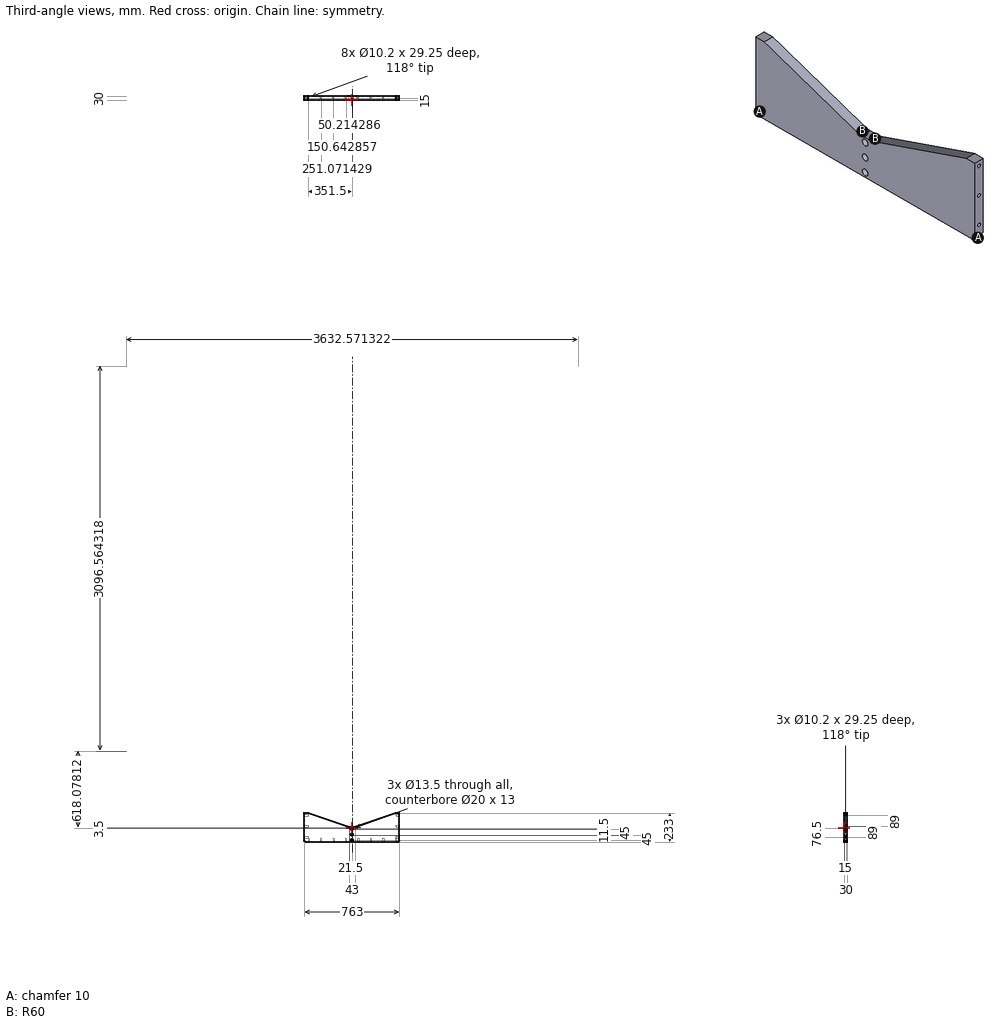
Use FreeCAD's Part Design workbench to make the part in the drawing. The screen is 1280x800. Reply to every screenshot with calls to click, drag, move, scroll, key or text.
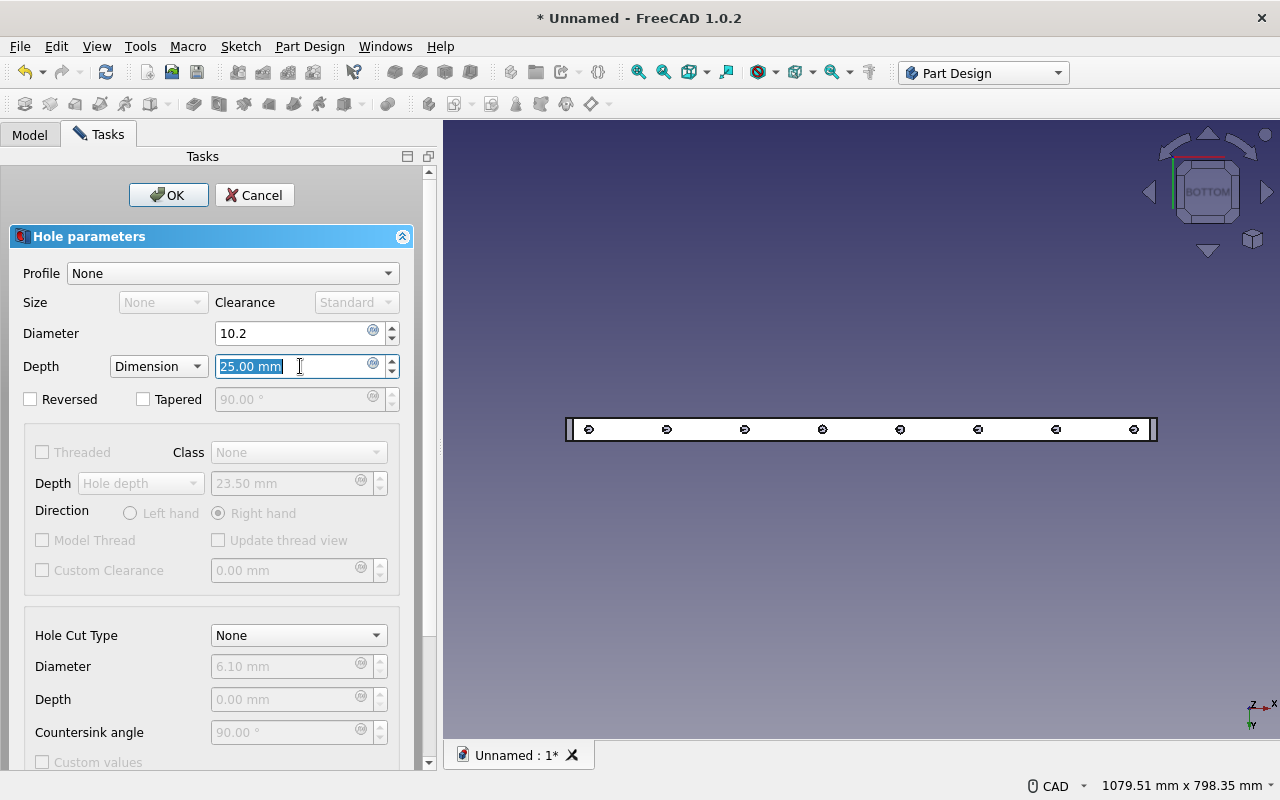
text(29.25)
key(Tab)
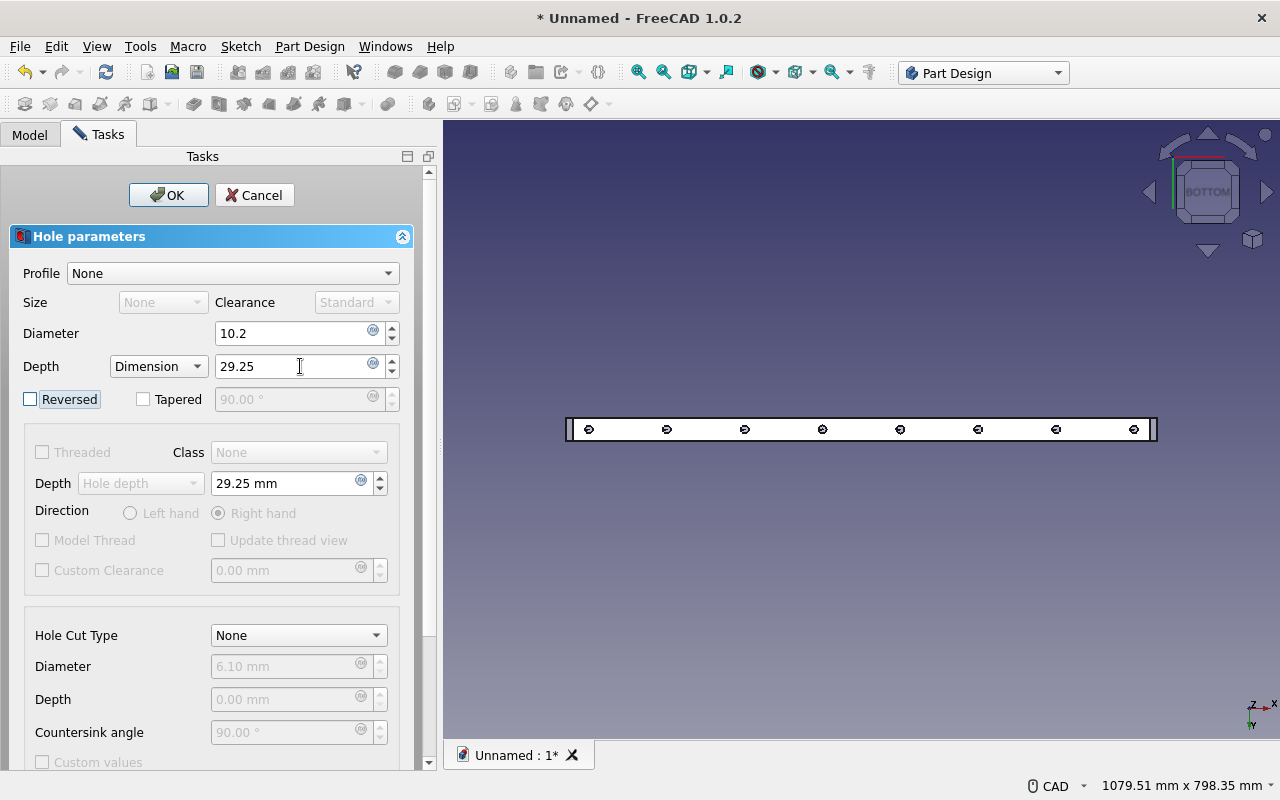
click(169, 195)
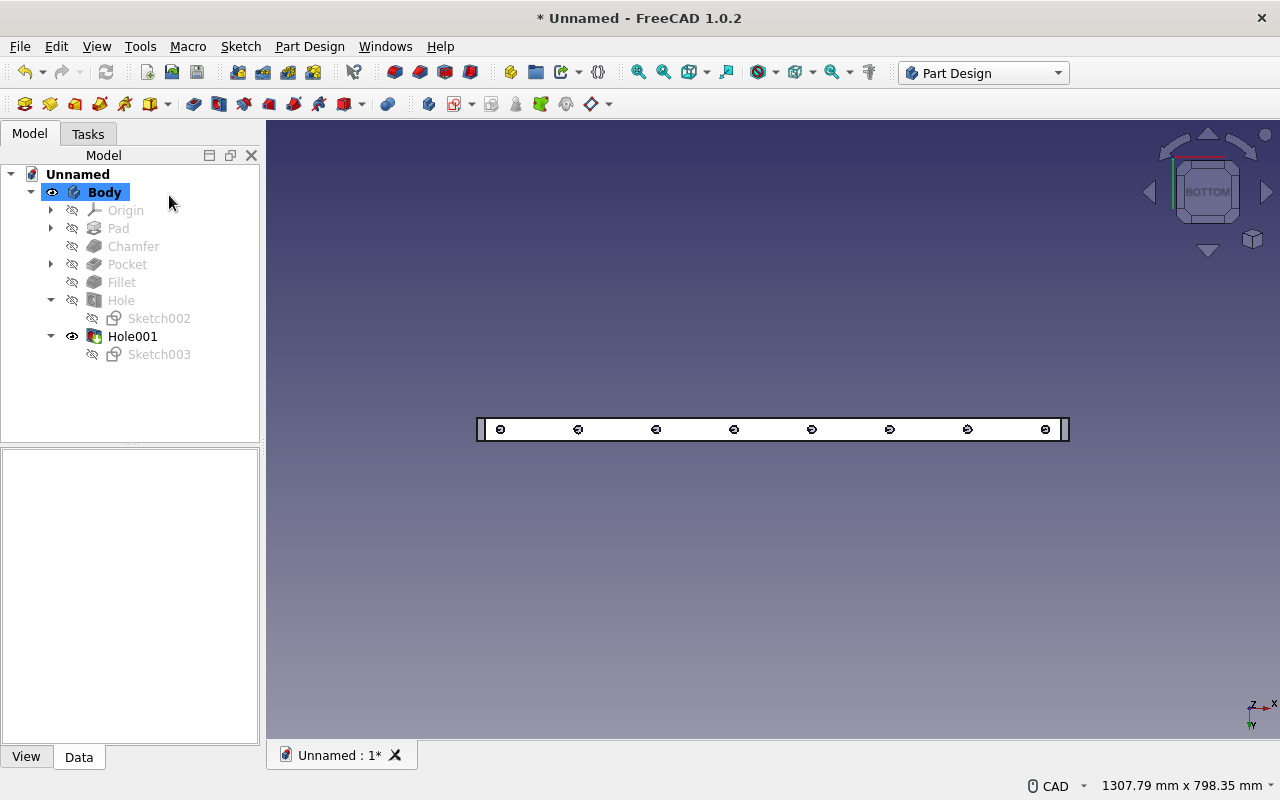
key(6)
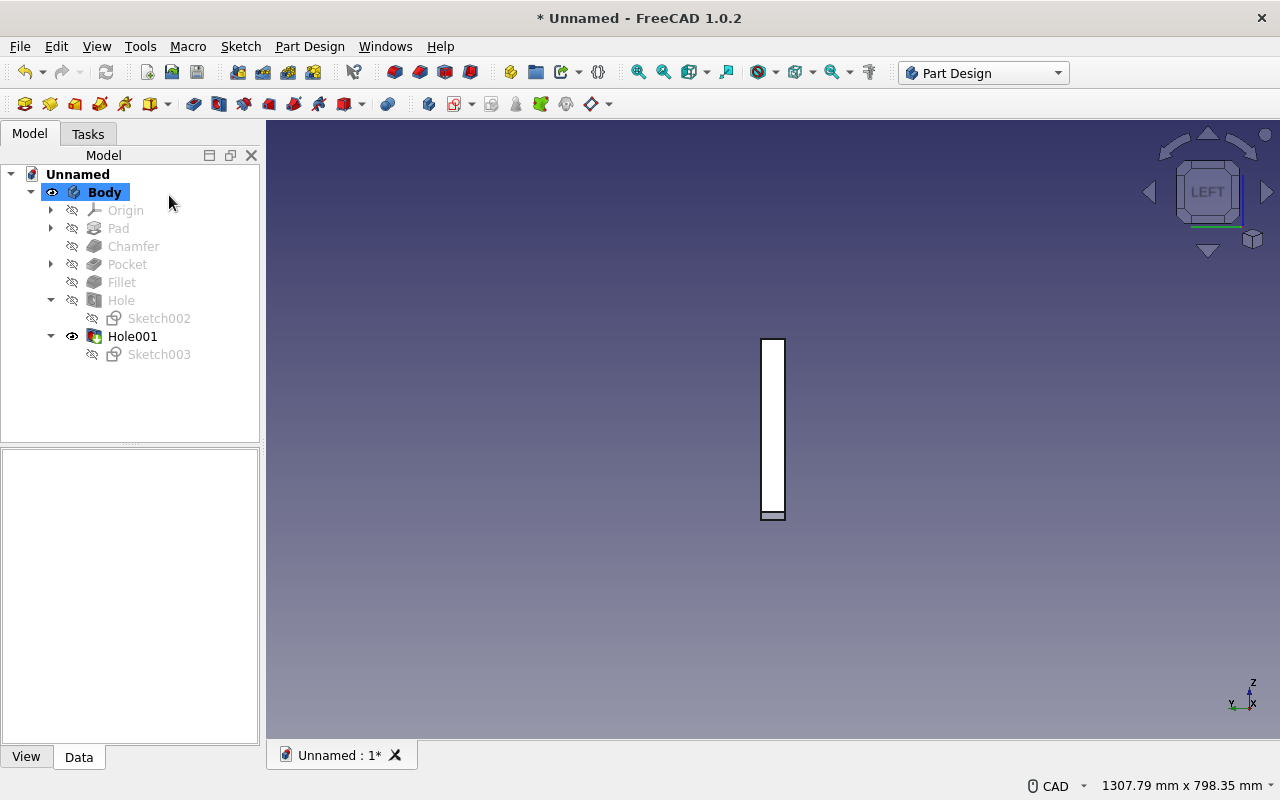
key(v)
key(f)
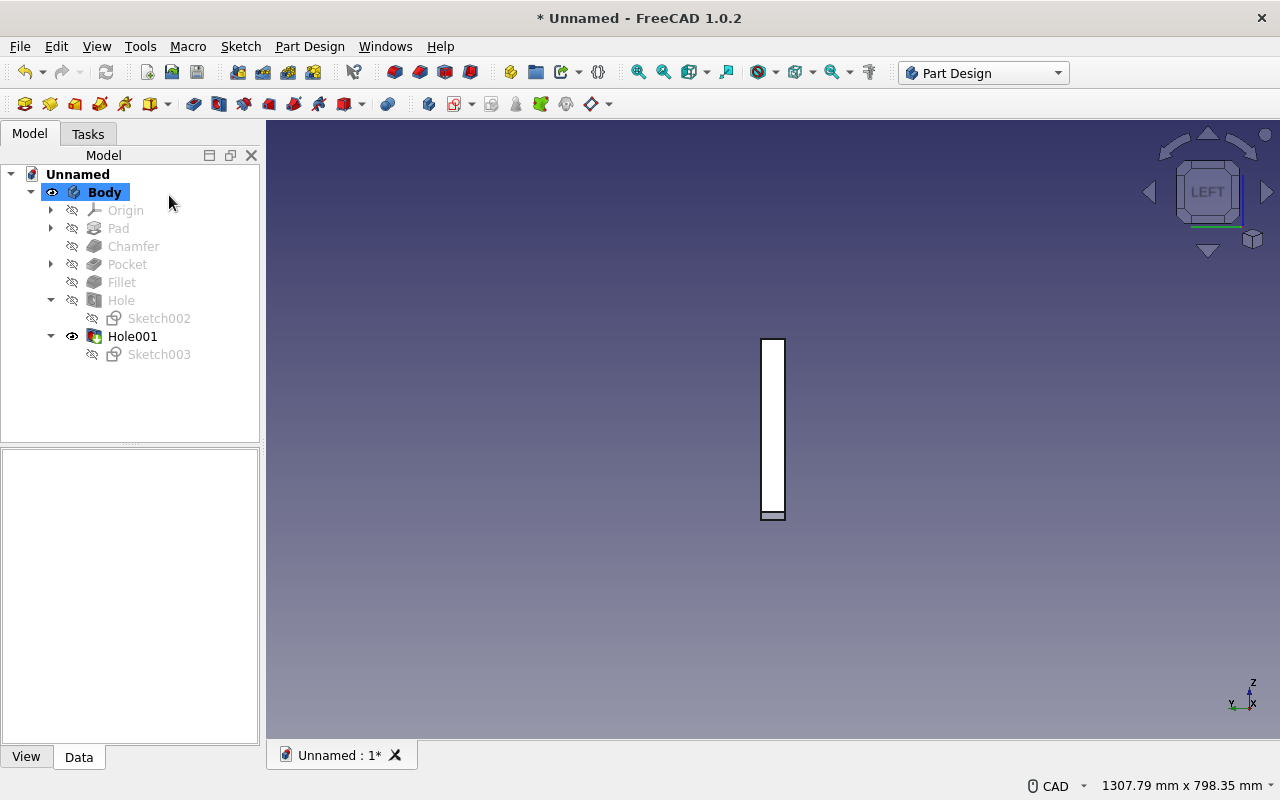
click(773, 474)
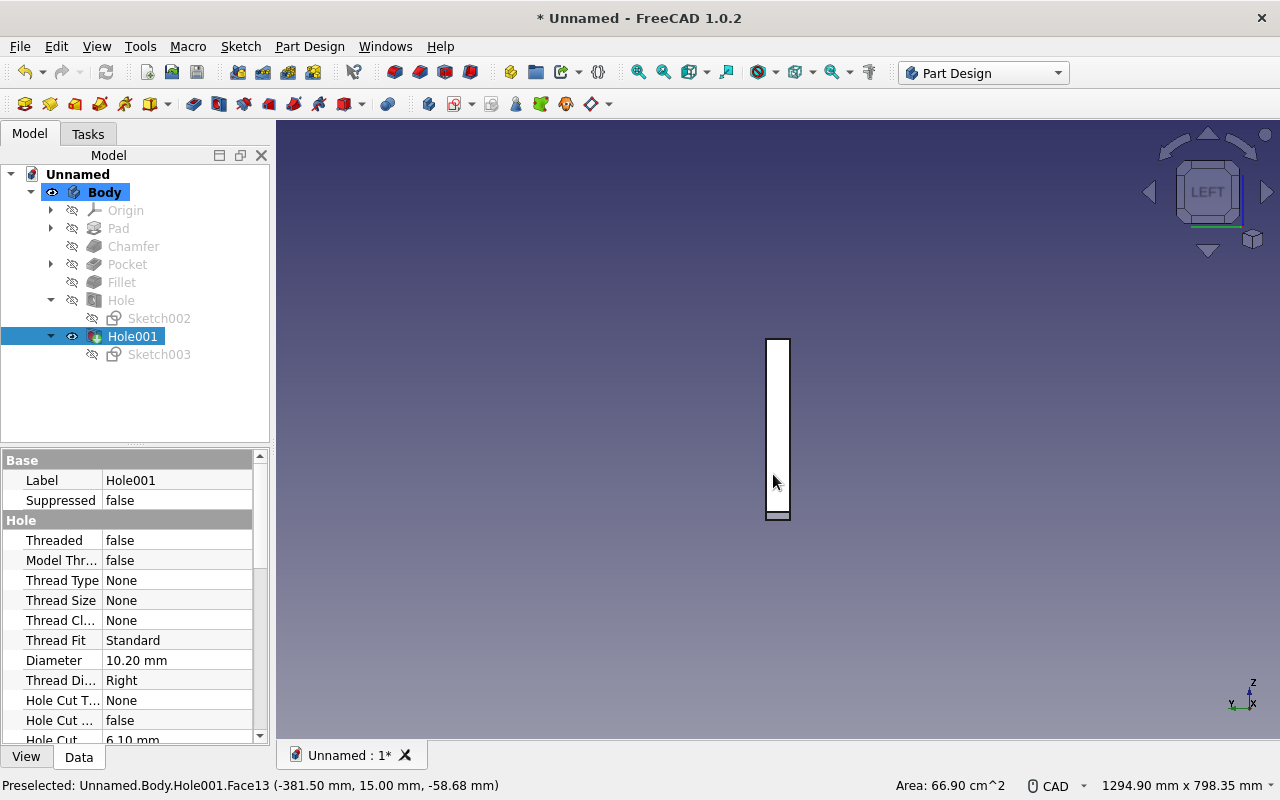
click(454, 104)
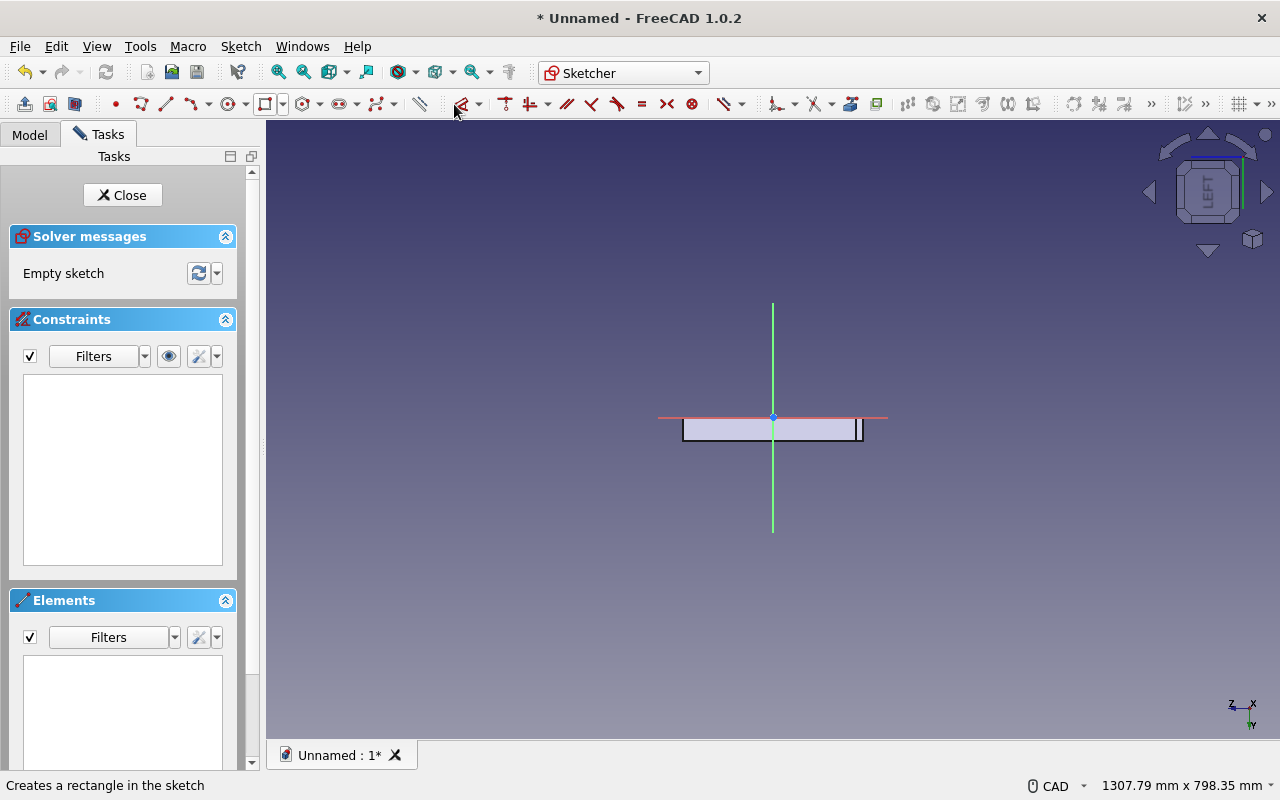
scroll(783, 424, up, 7)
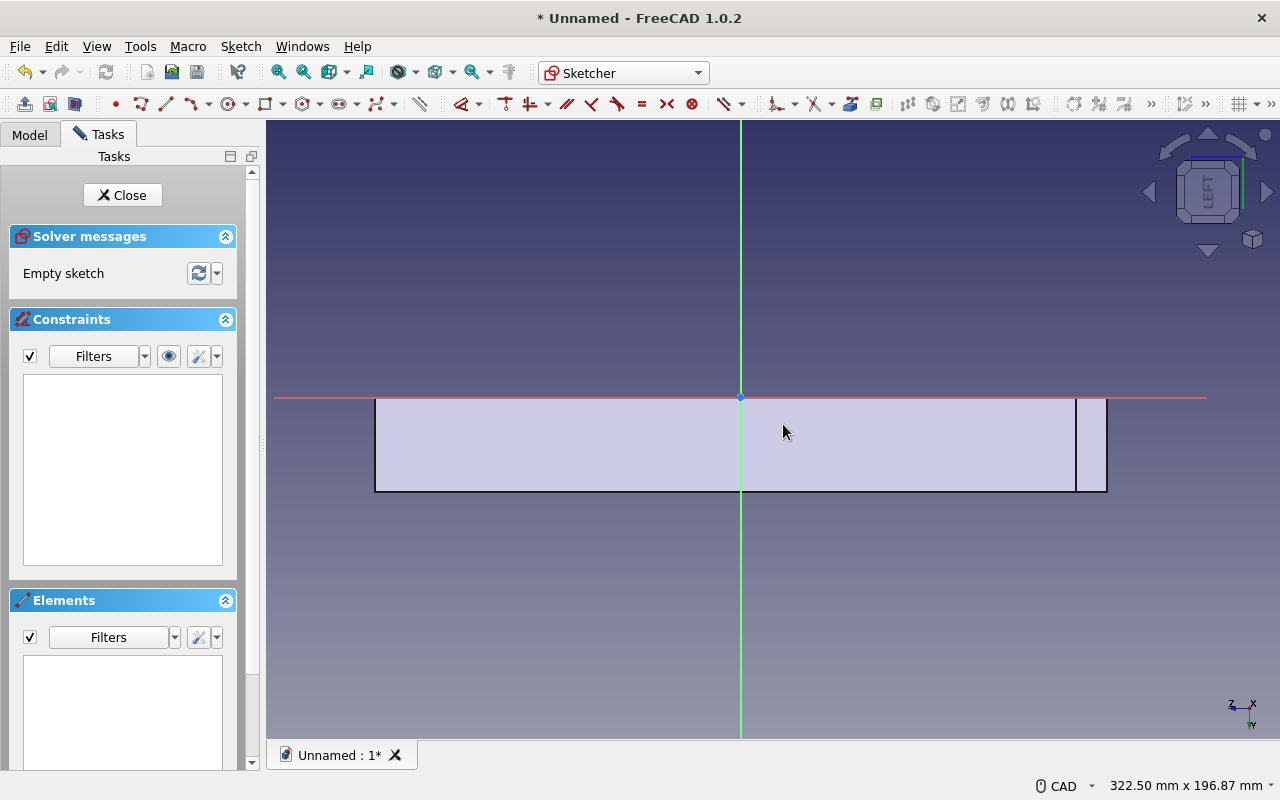
key(g)
key(c)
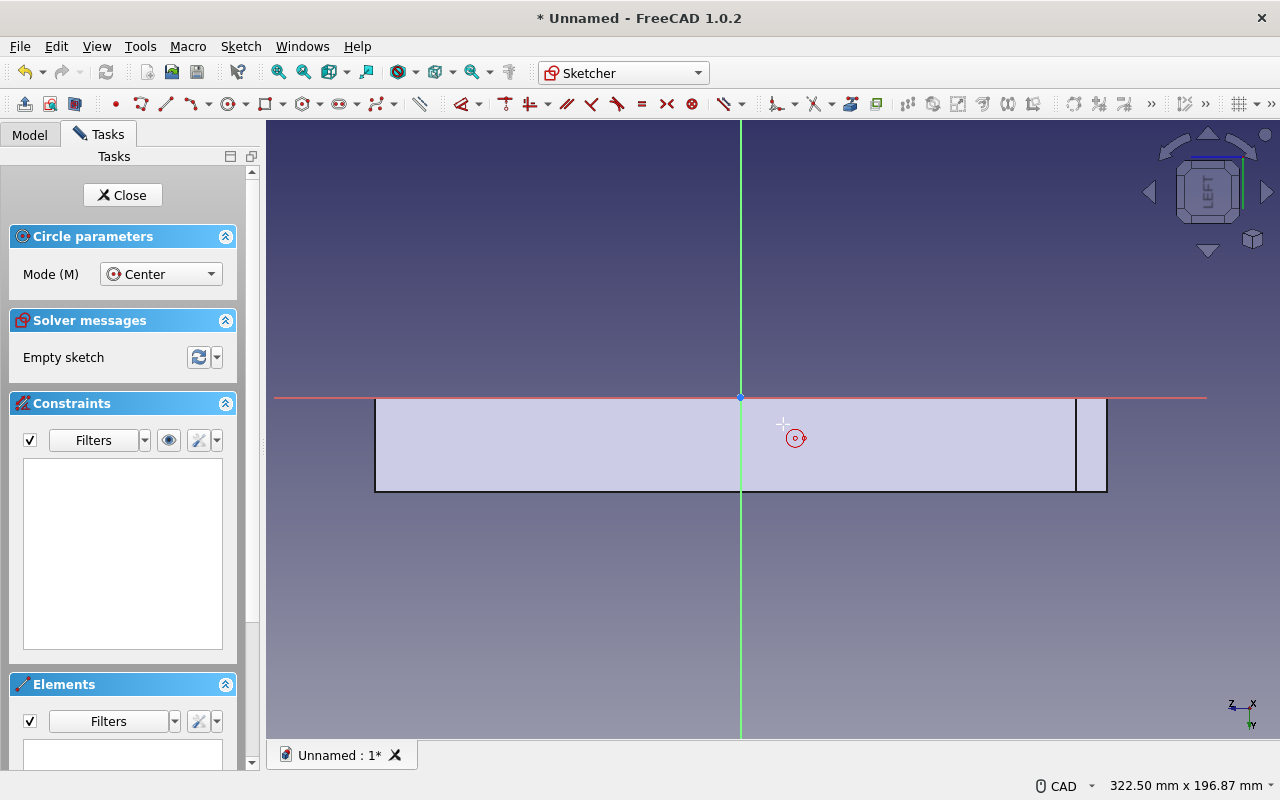
scroll(981, 445, up, 2)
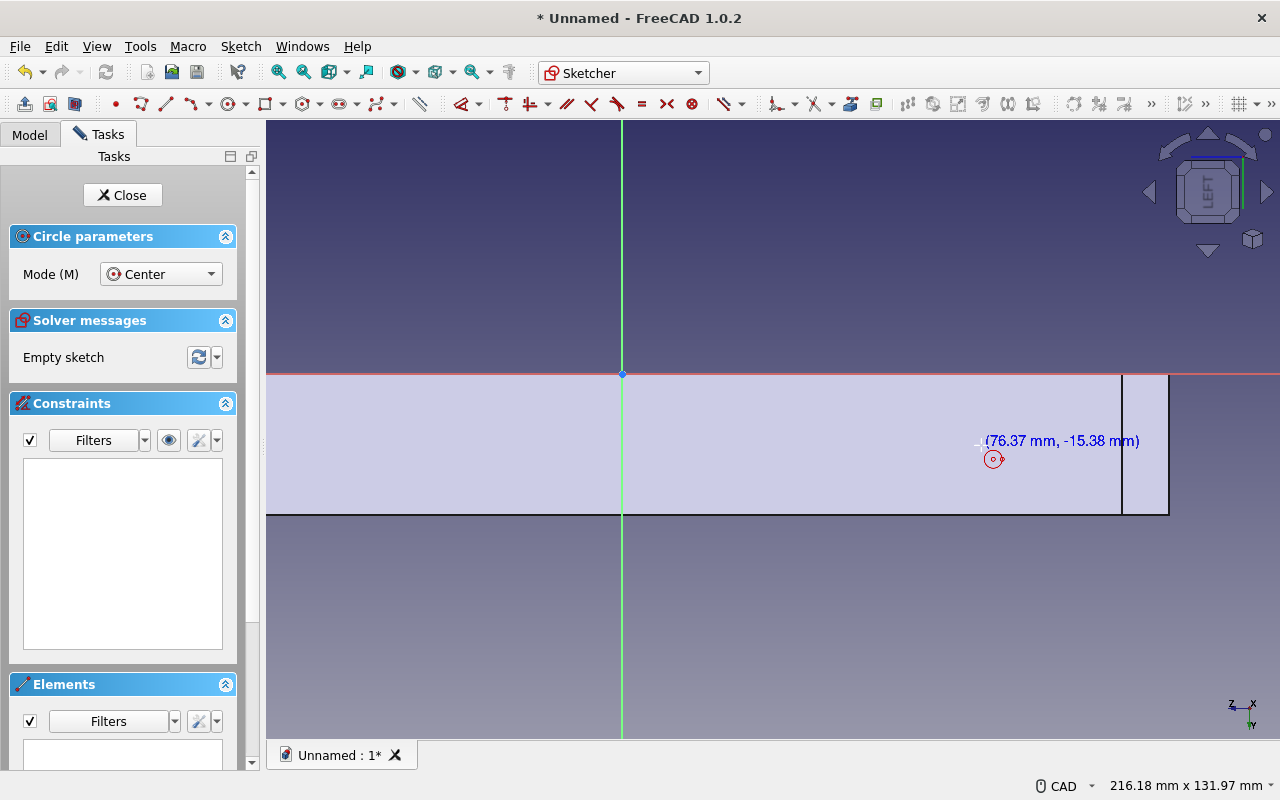
click(981, 444)
click(998, 428)